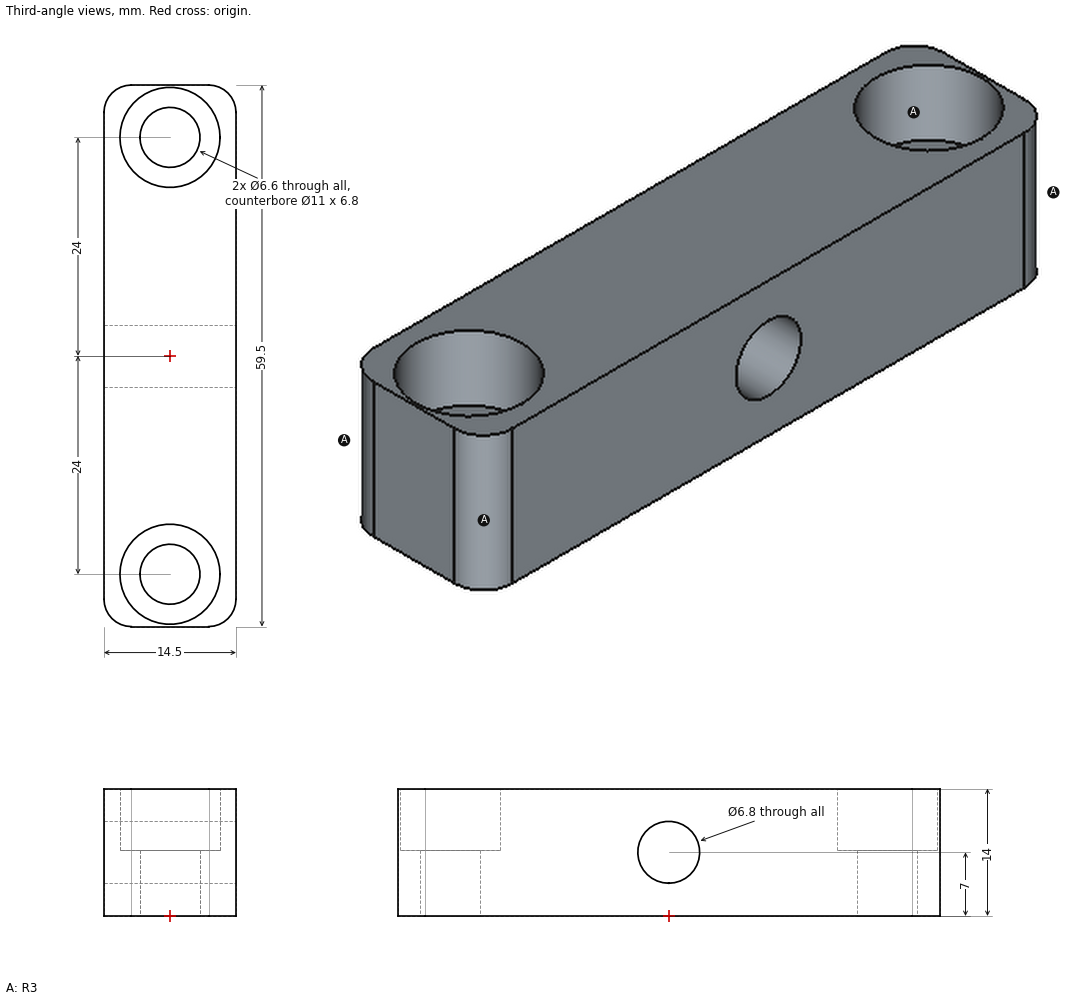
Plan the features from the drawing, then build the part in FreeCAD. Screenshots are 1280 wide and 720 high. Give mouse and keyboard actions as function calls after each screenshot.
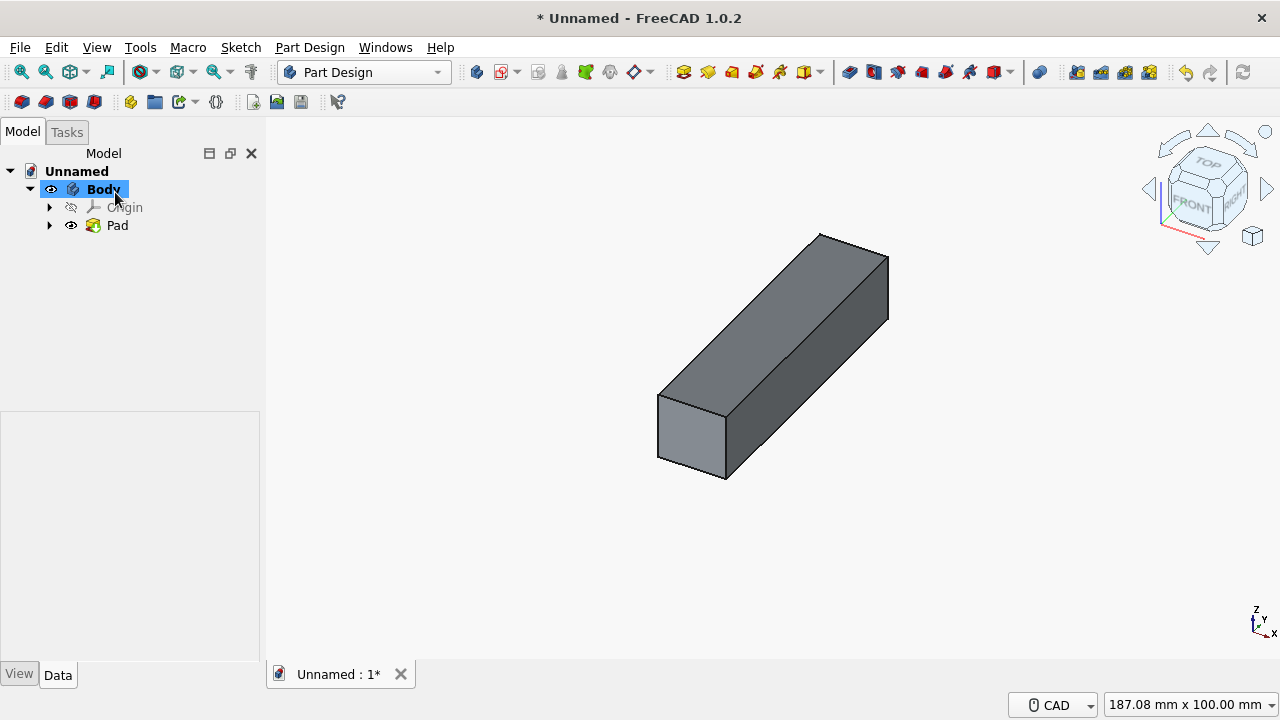
click(726, 447)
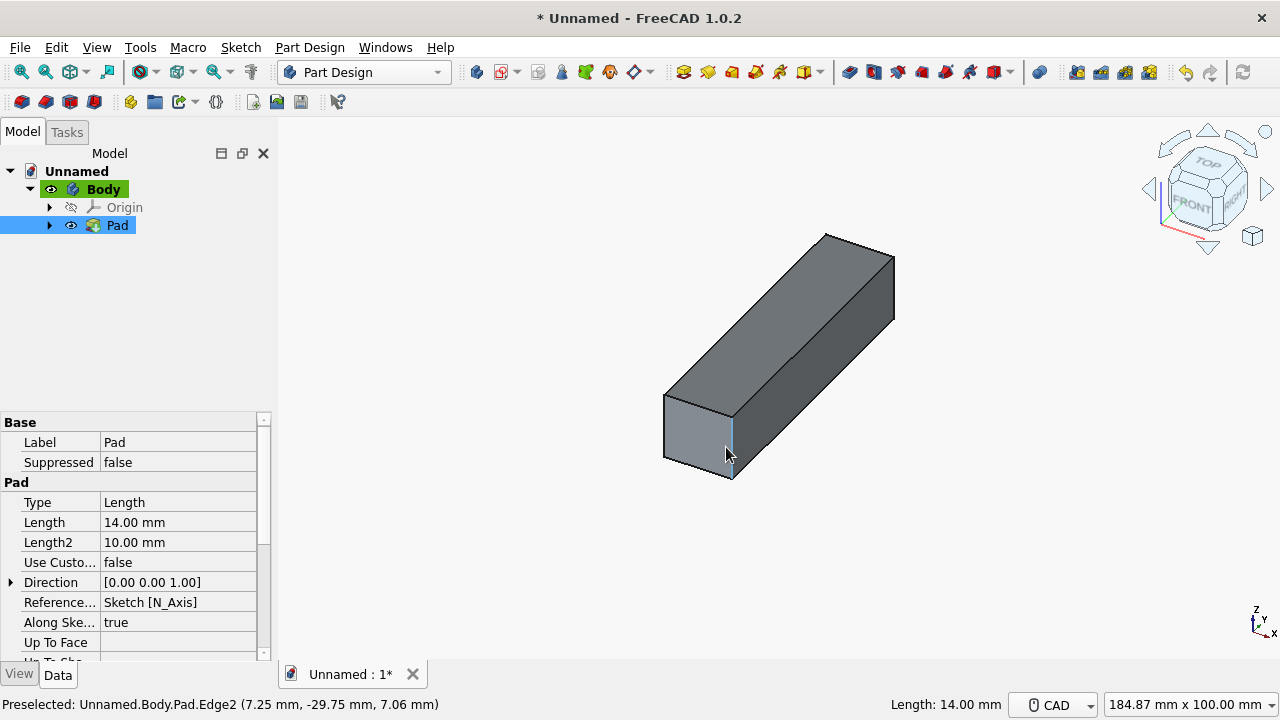
key(0)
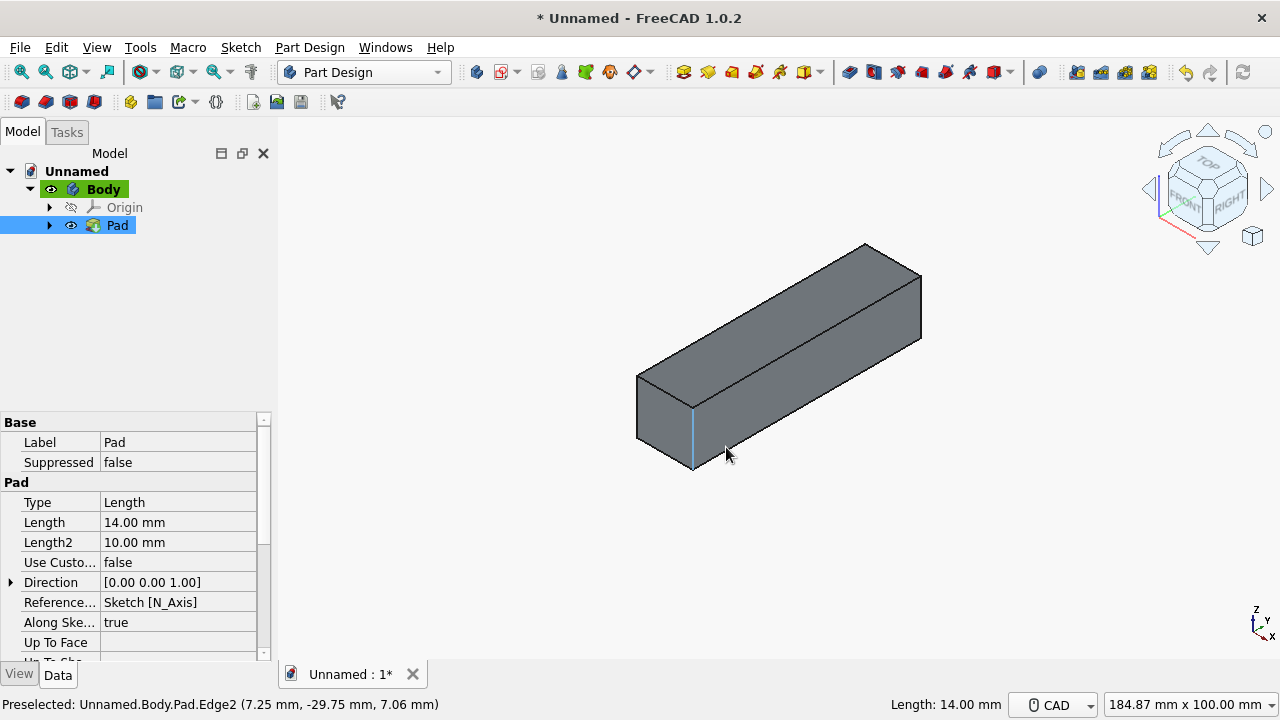
key(v)
key(f)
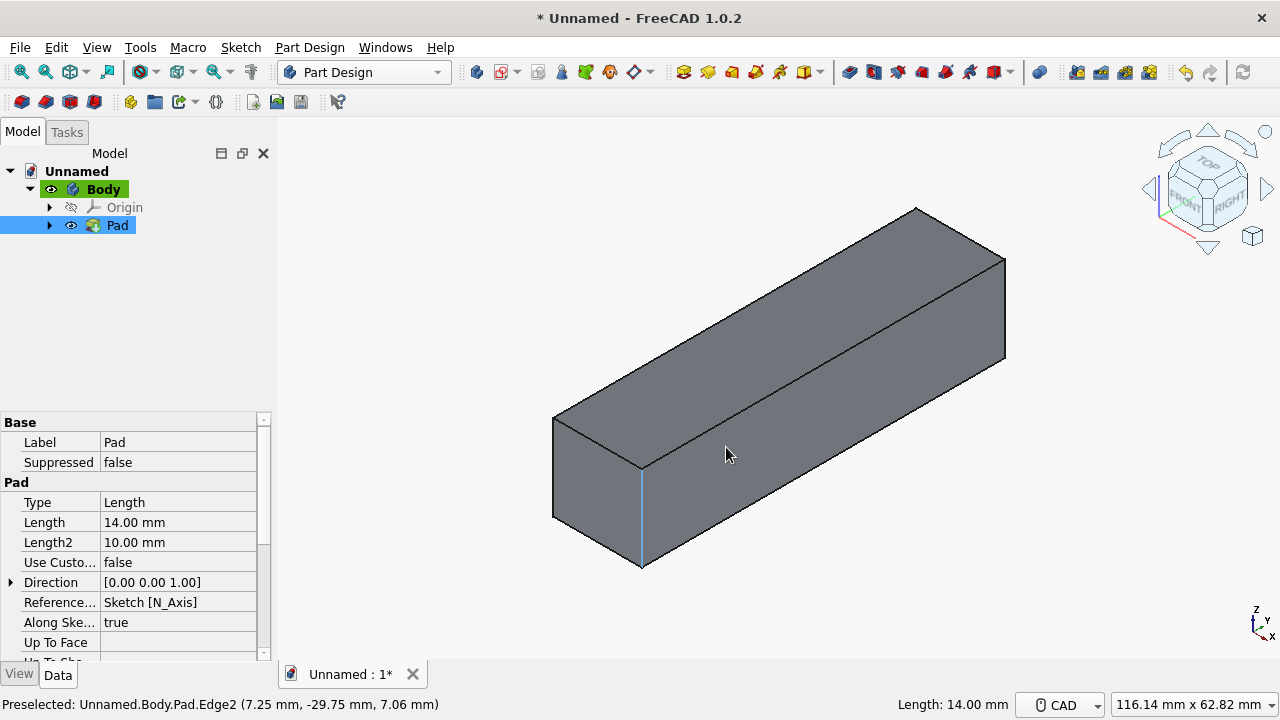
key(2)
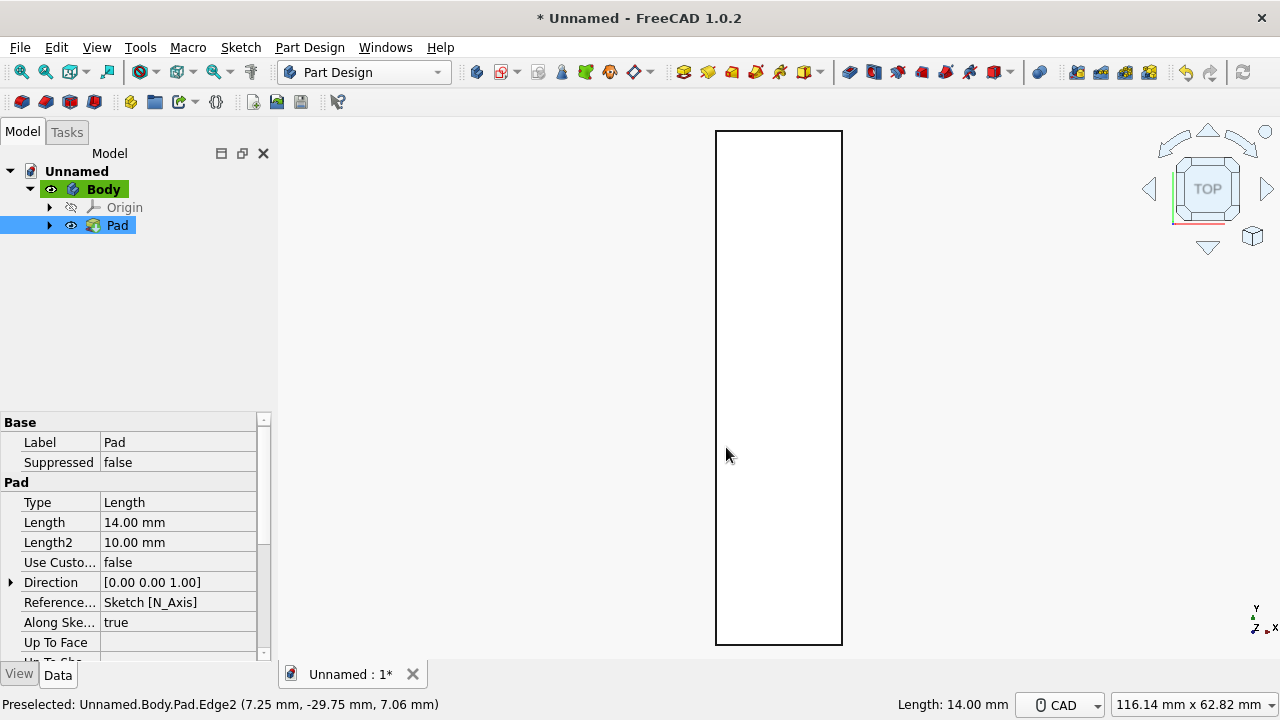
key(1)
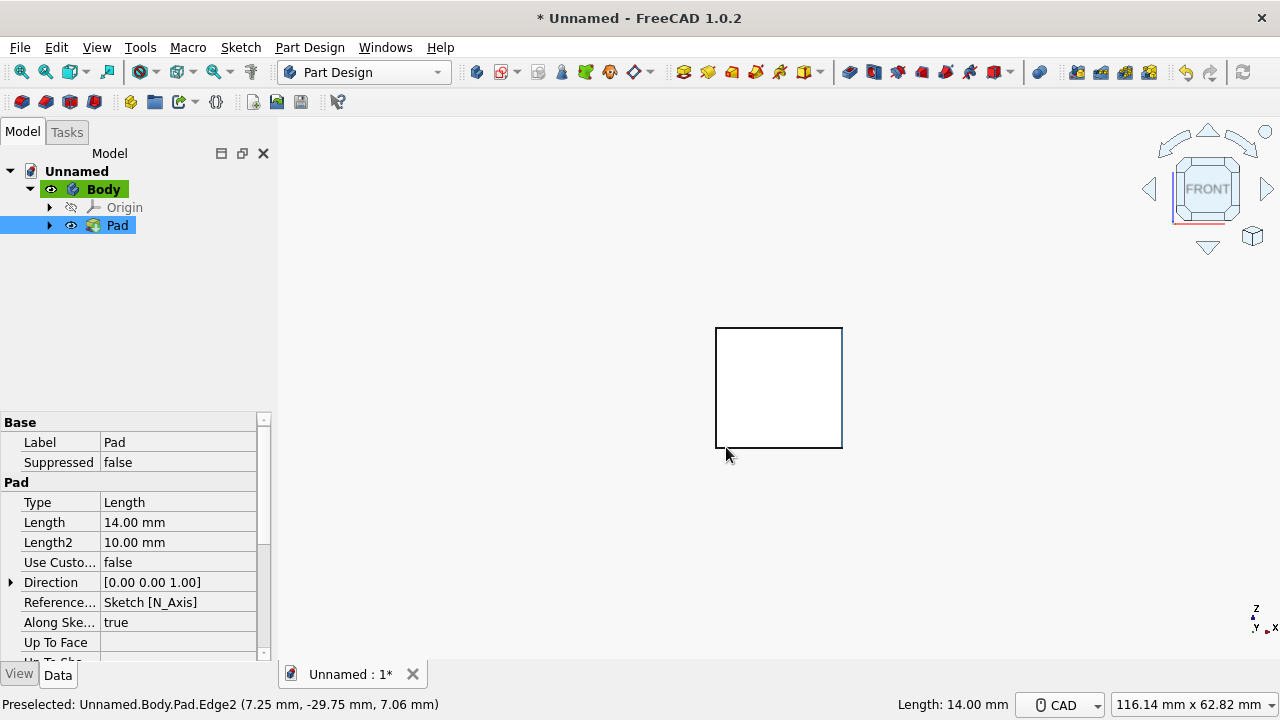
click(22, 72)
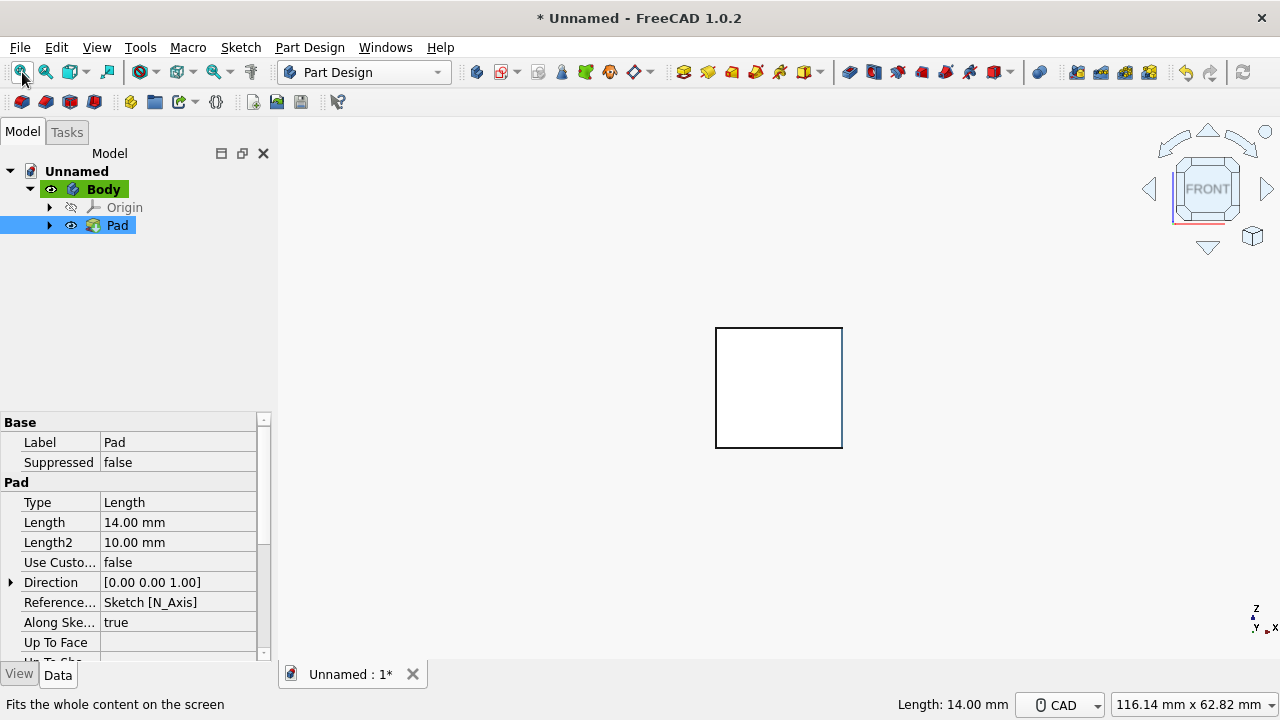
click(716, 387, ctrl)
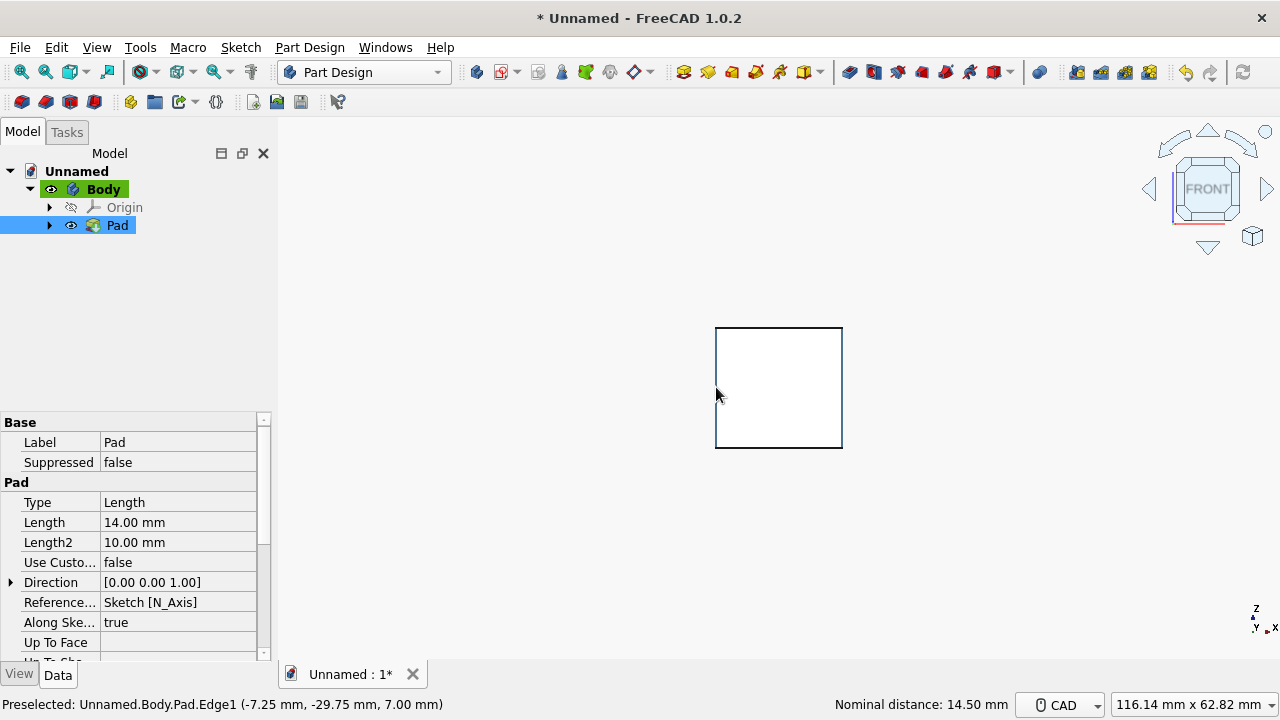
key(3)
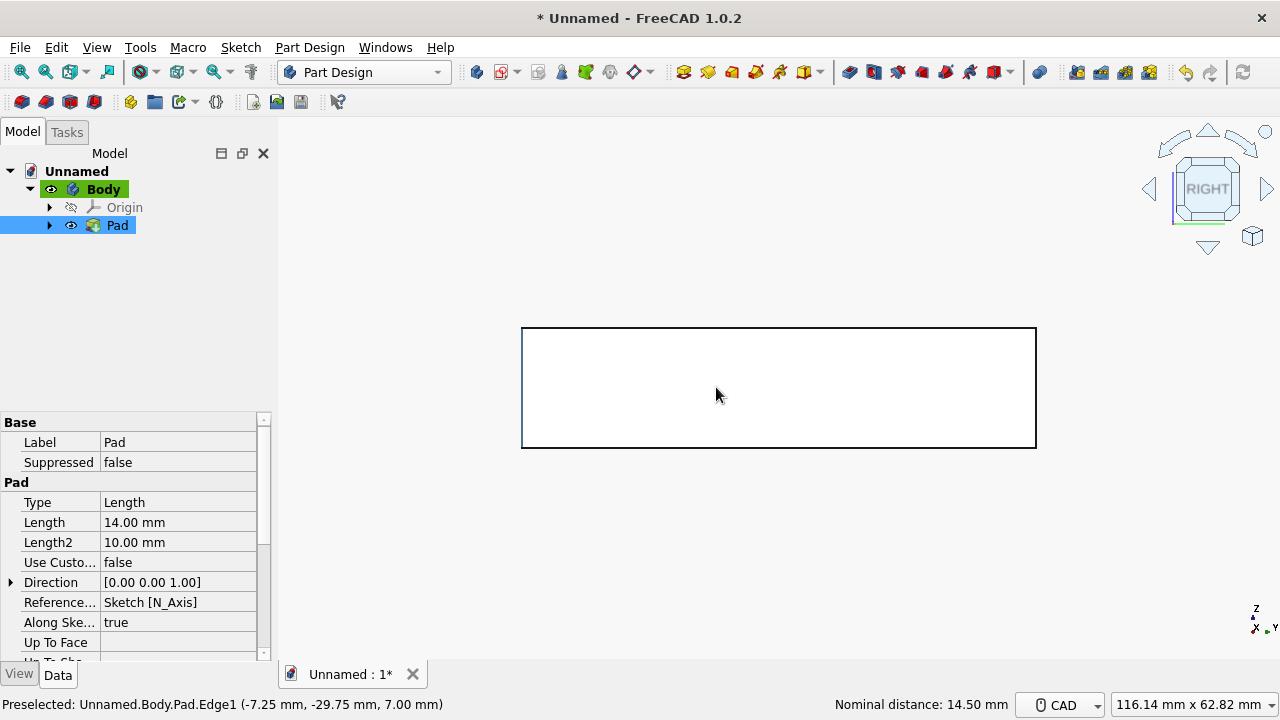
click(1036, 387, ctrl)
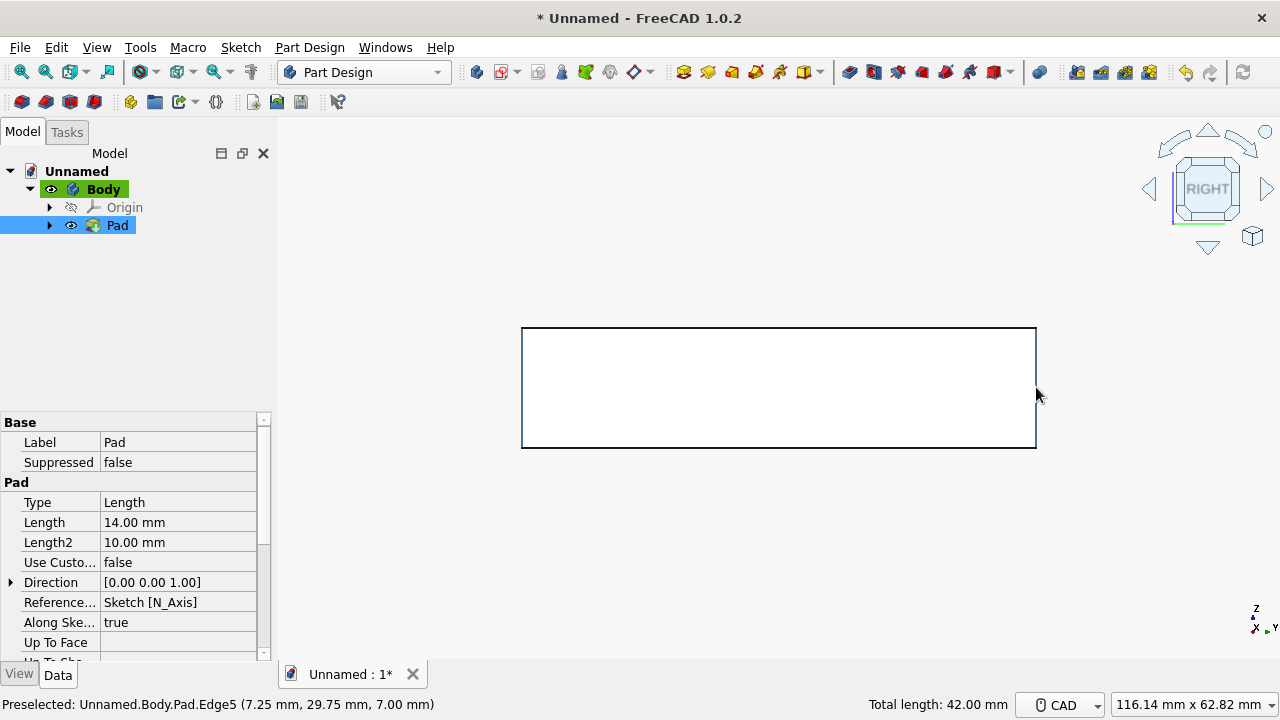
key(5)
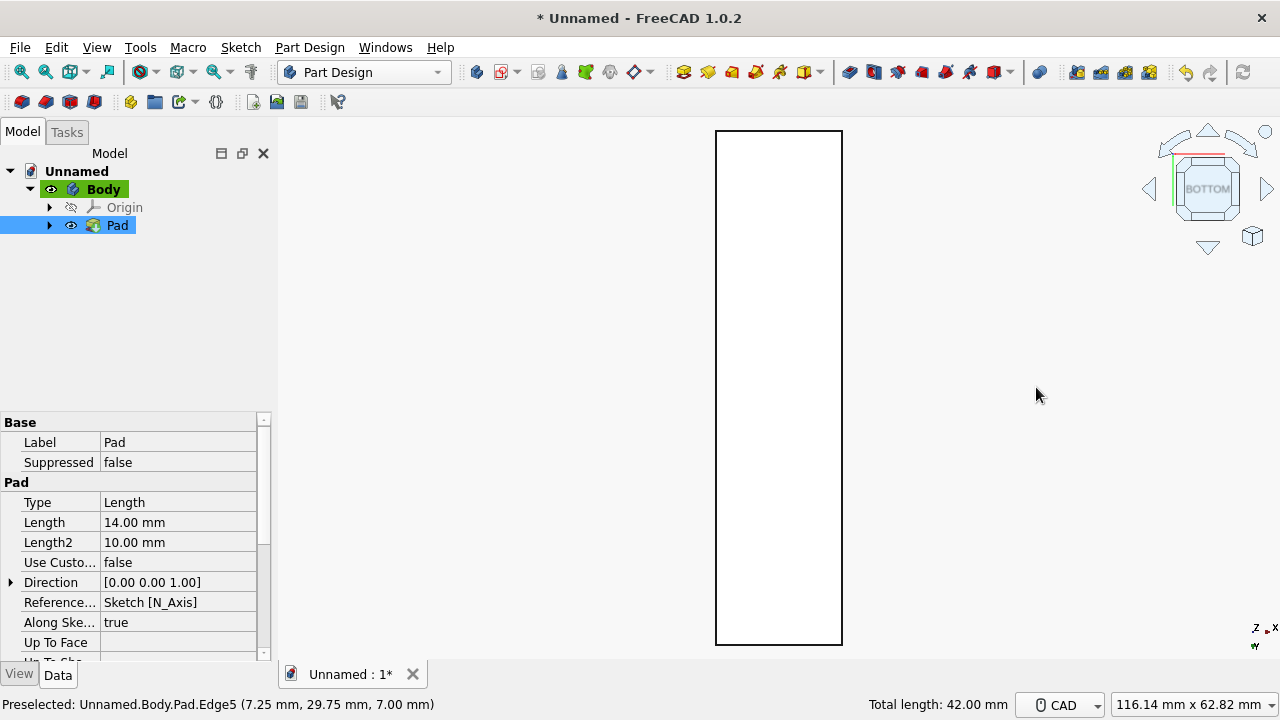
key(4)